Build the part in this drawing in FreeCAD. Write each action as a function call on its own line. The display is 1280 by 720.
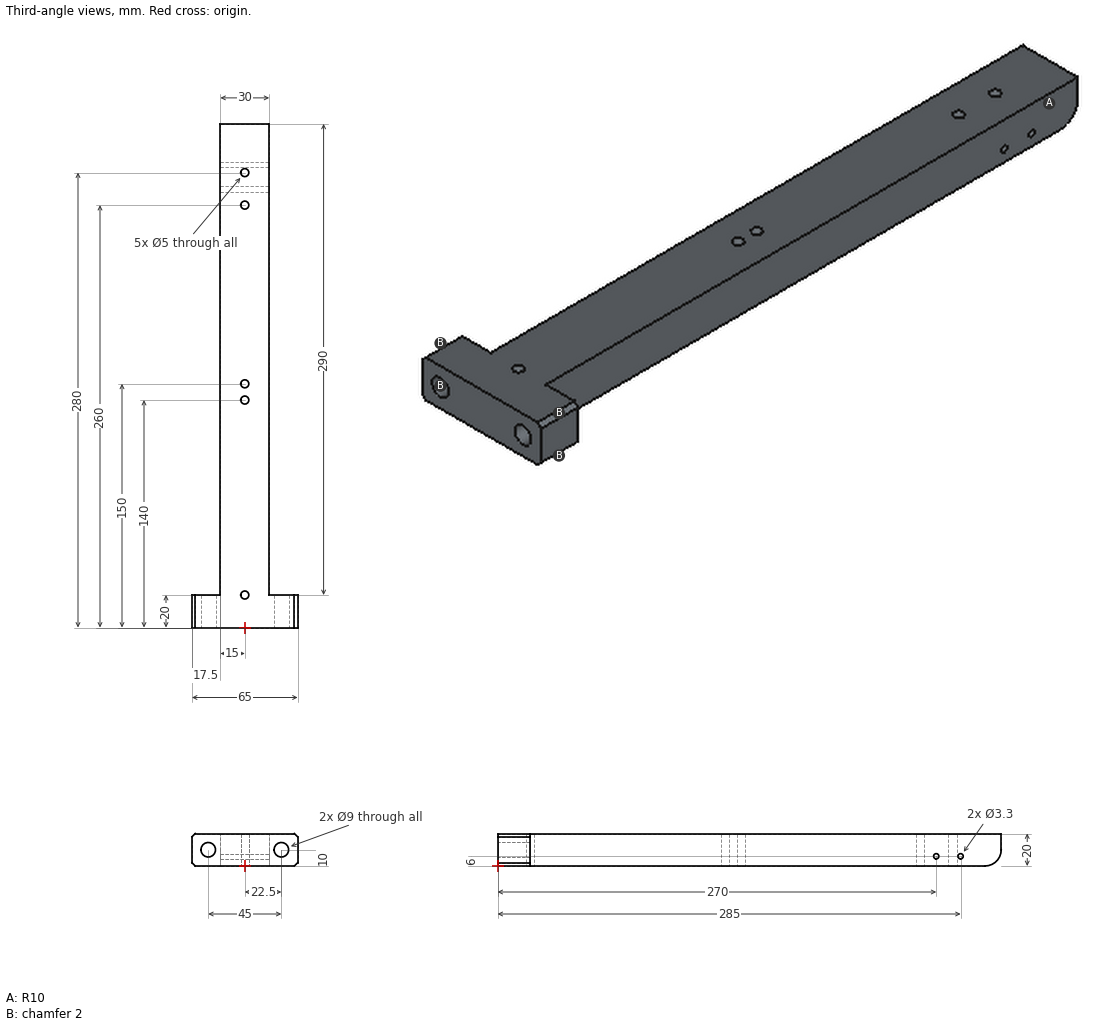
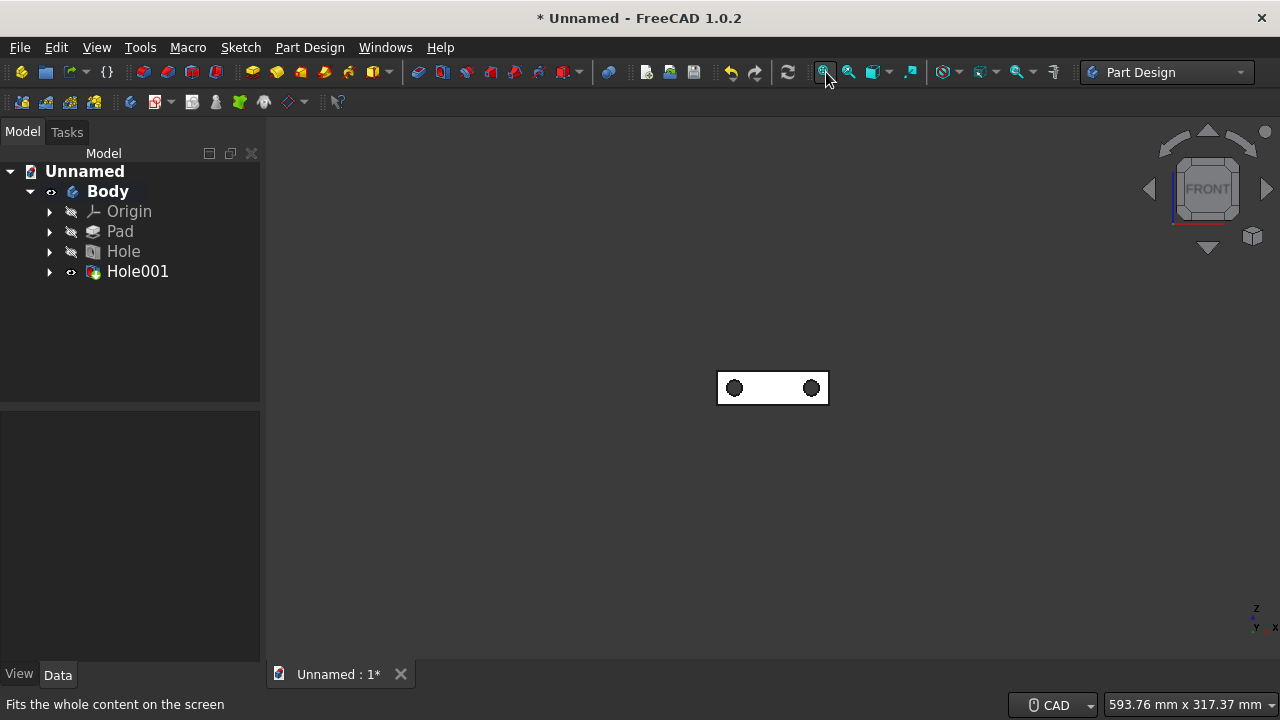
key(3)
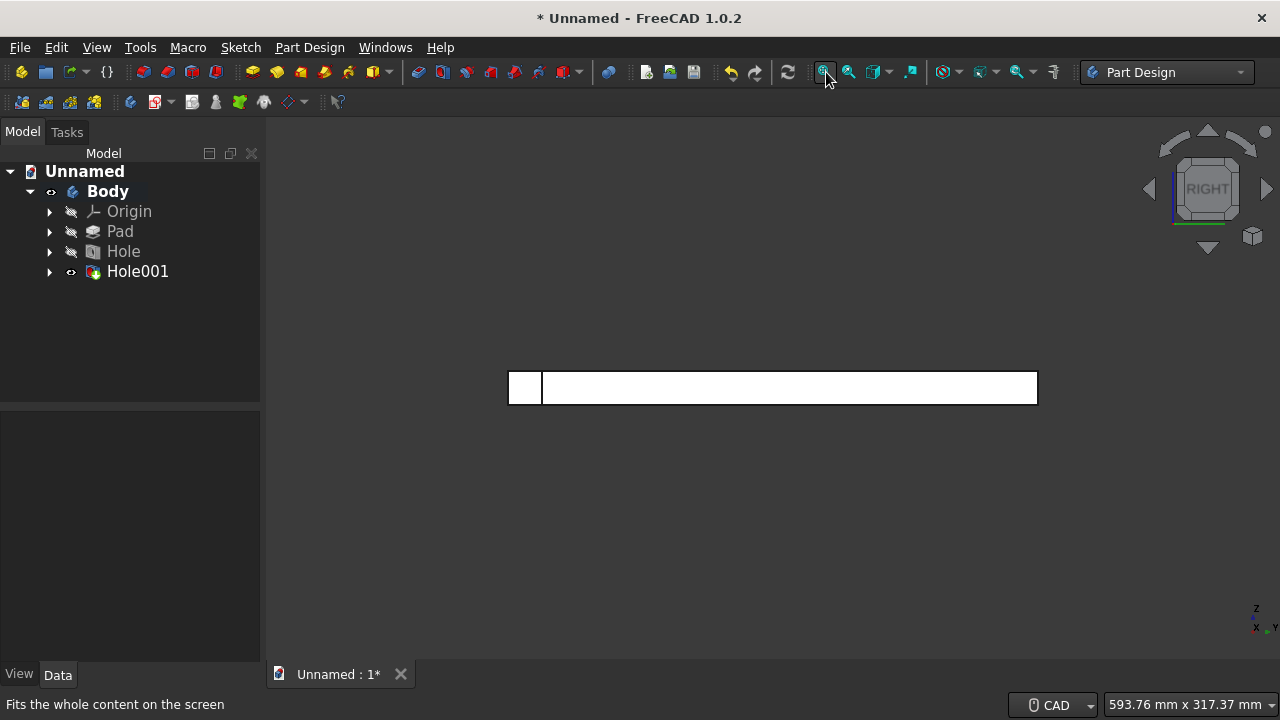
key(5)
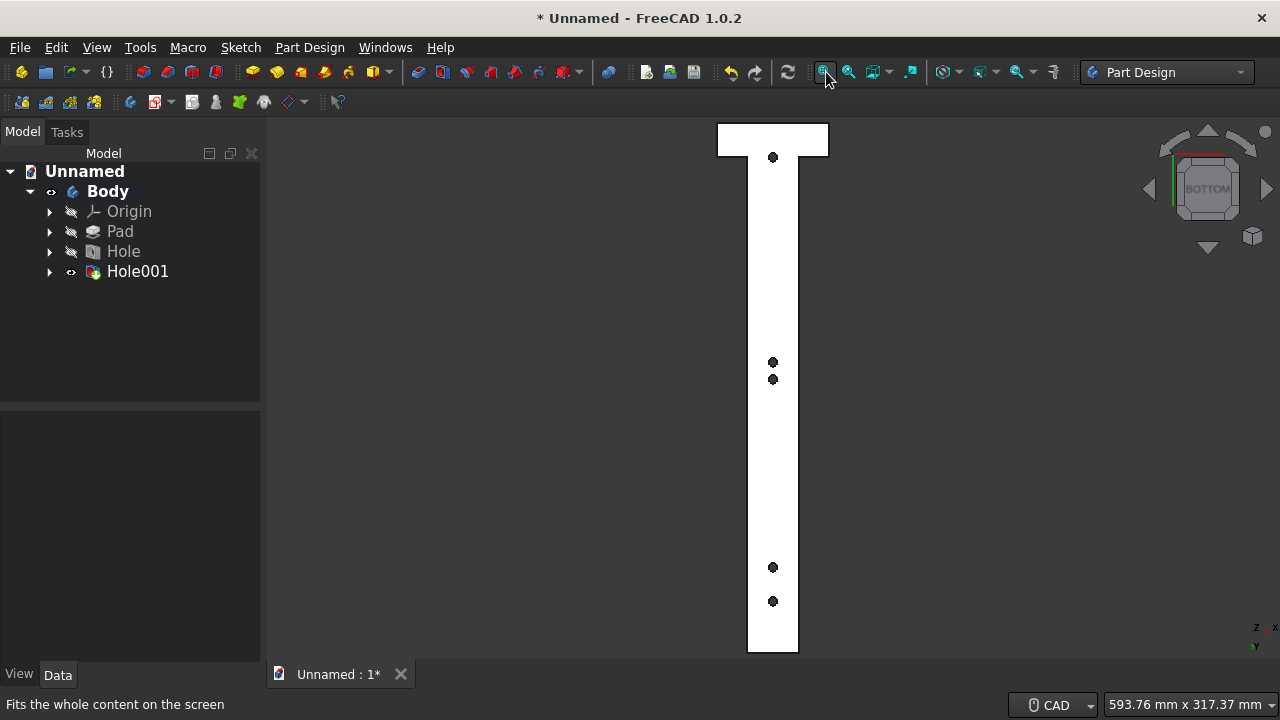
key(4)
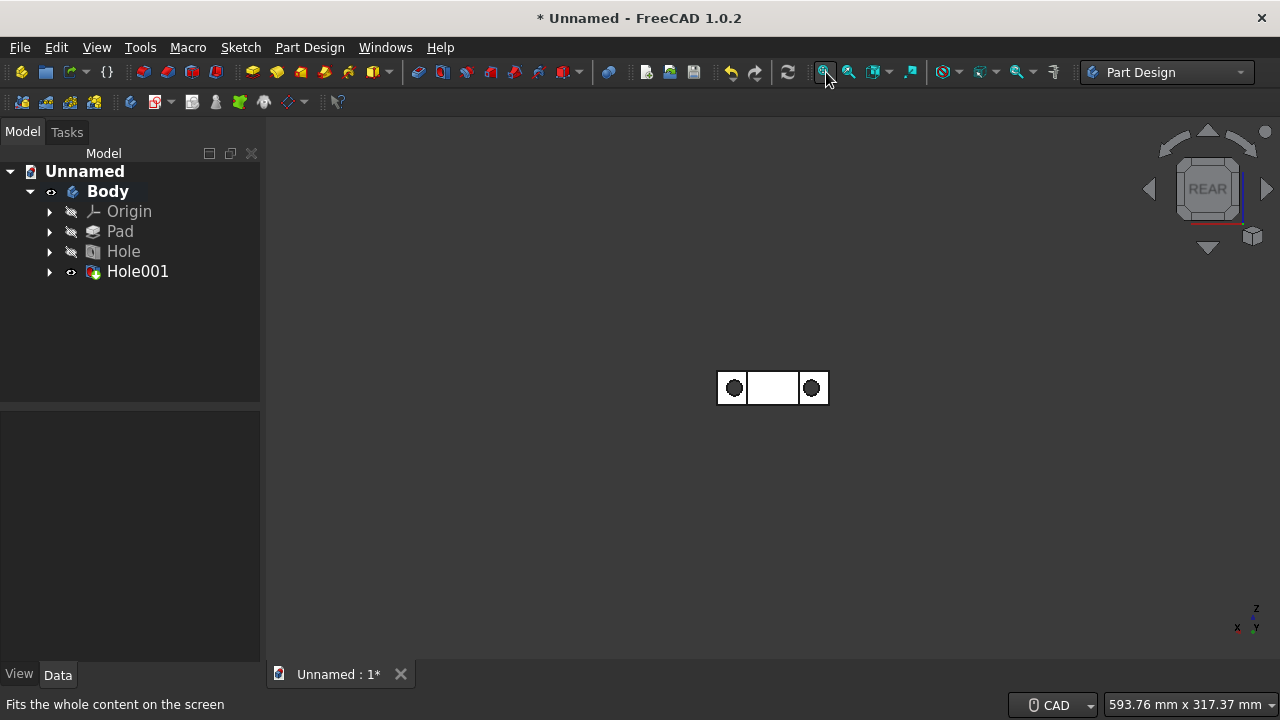
key(v)
key(f)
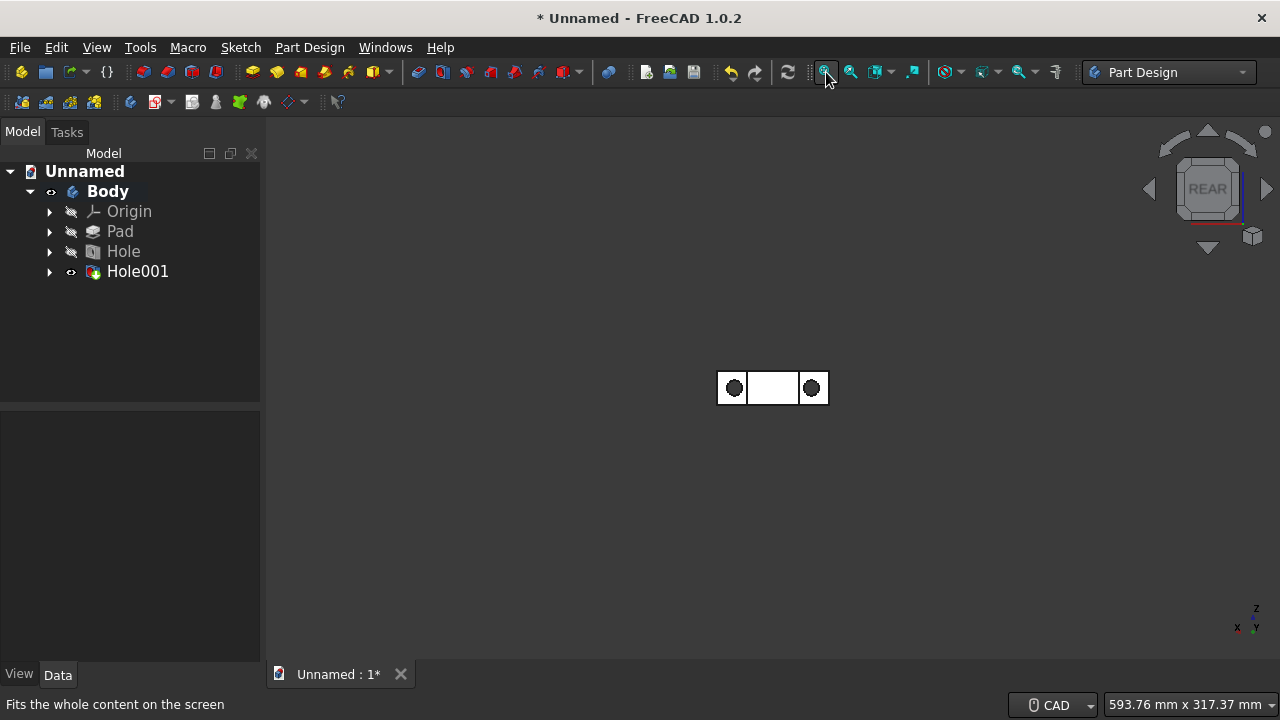
click(773, 404)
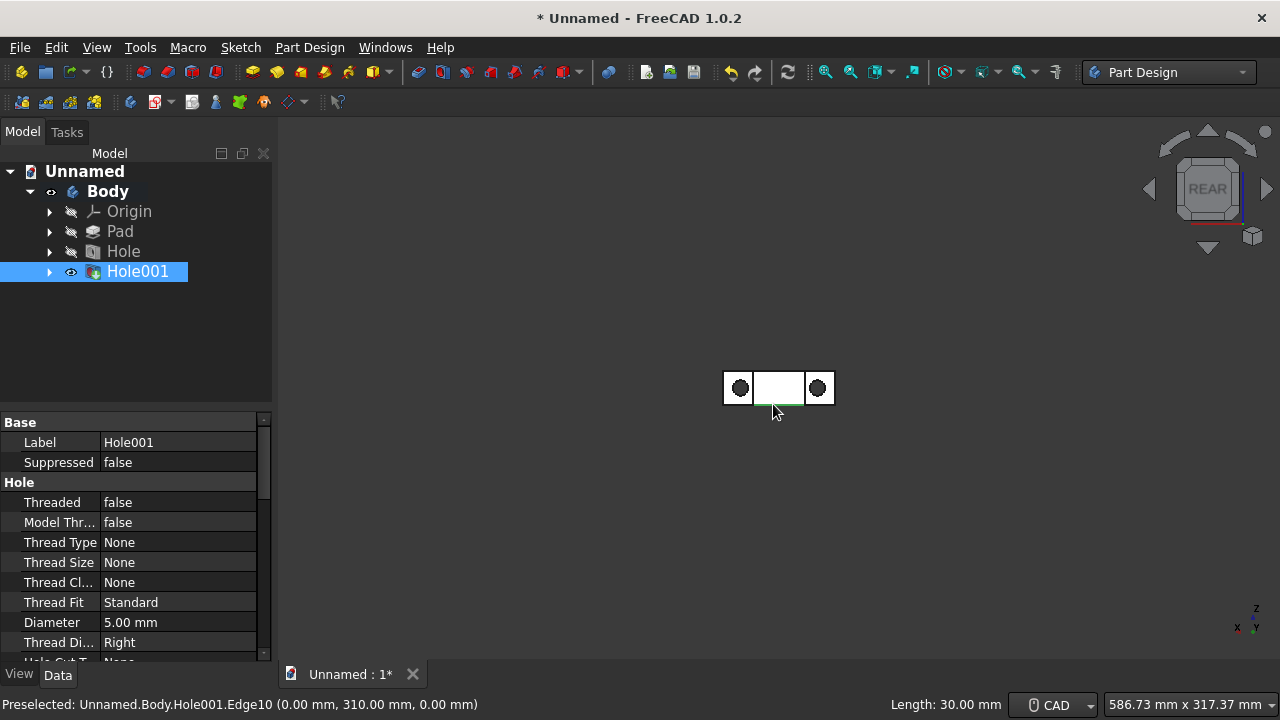
click(144, 72)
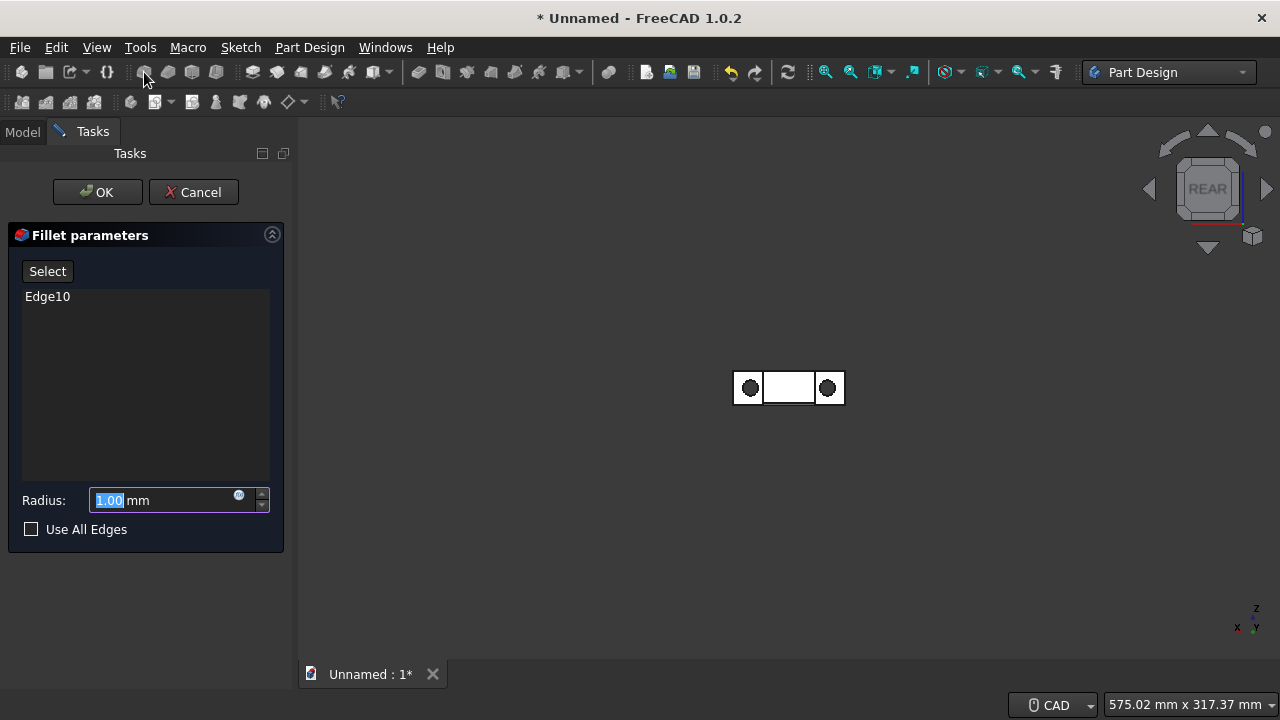
text(10)
key(Tab)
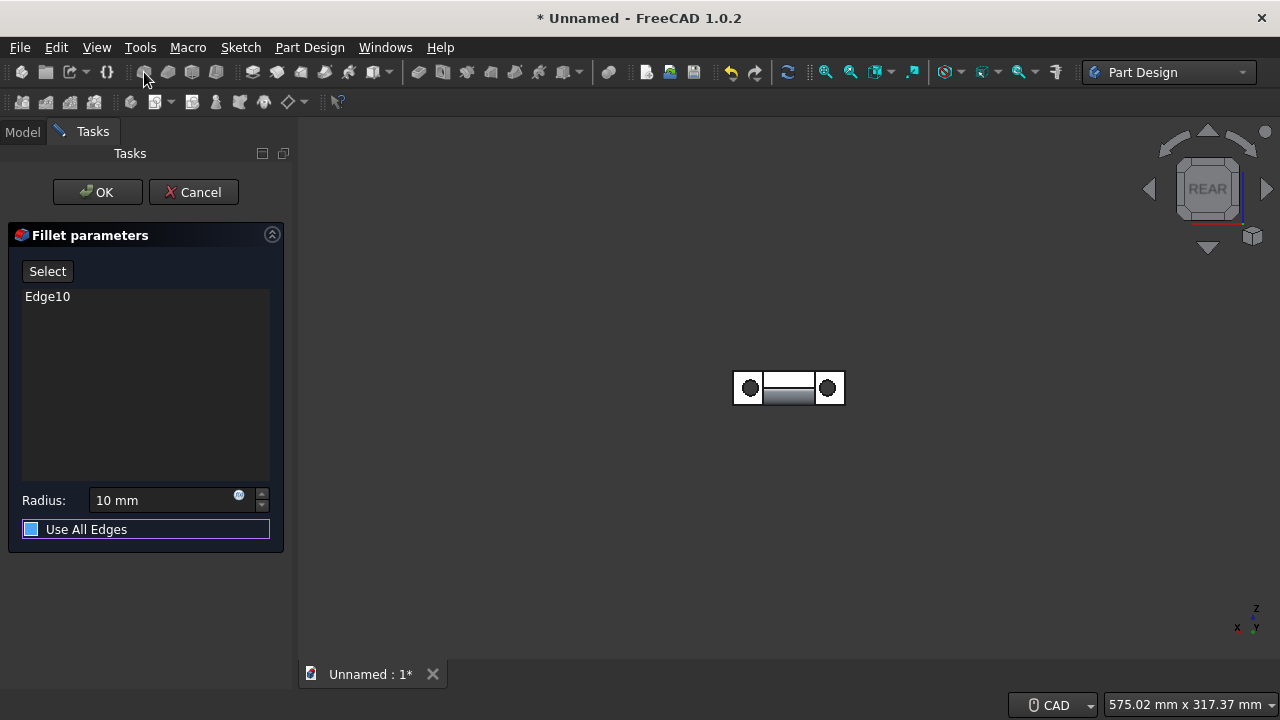
click(98, 192)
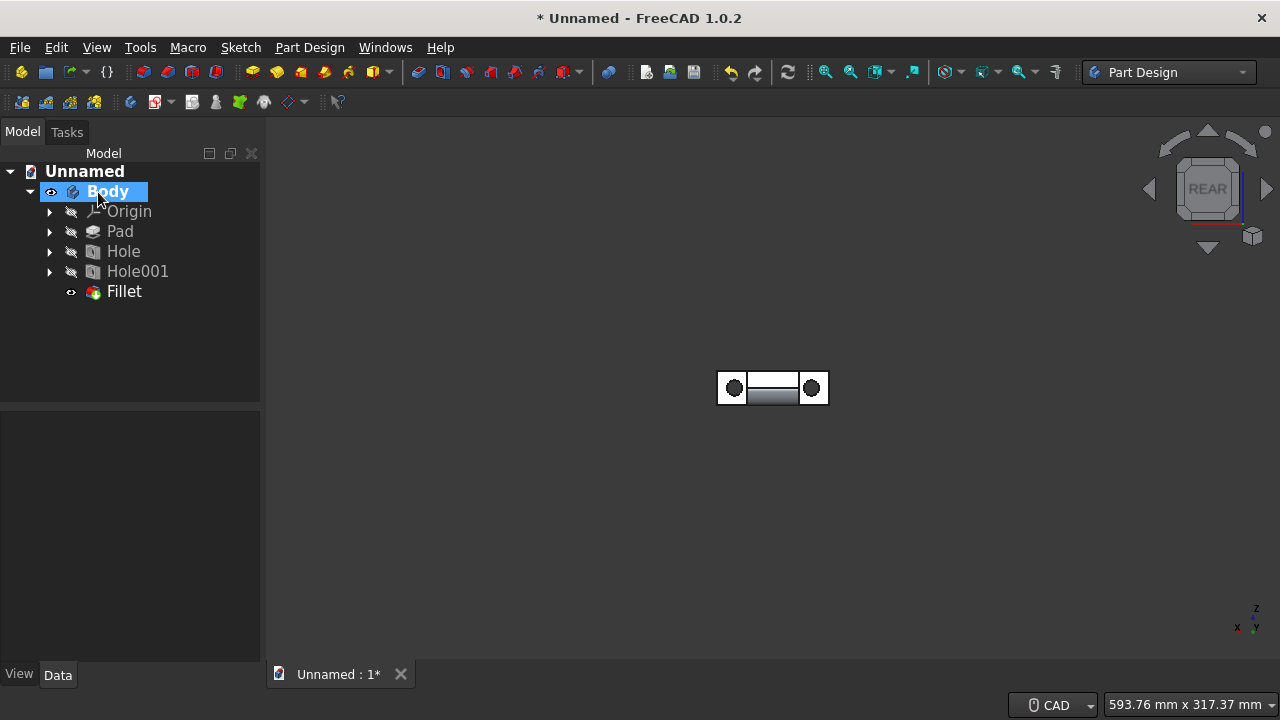
key(v)
key(f)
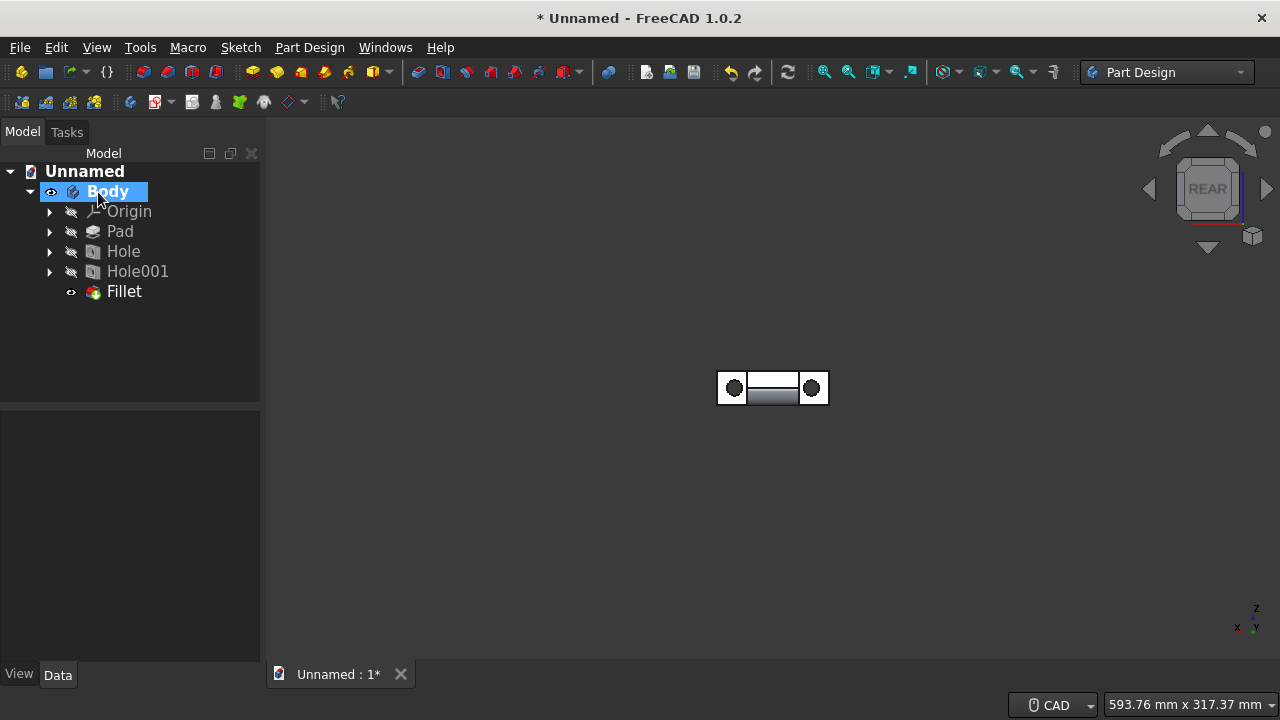
key(0)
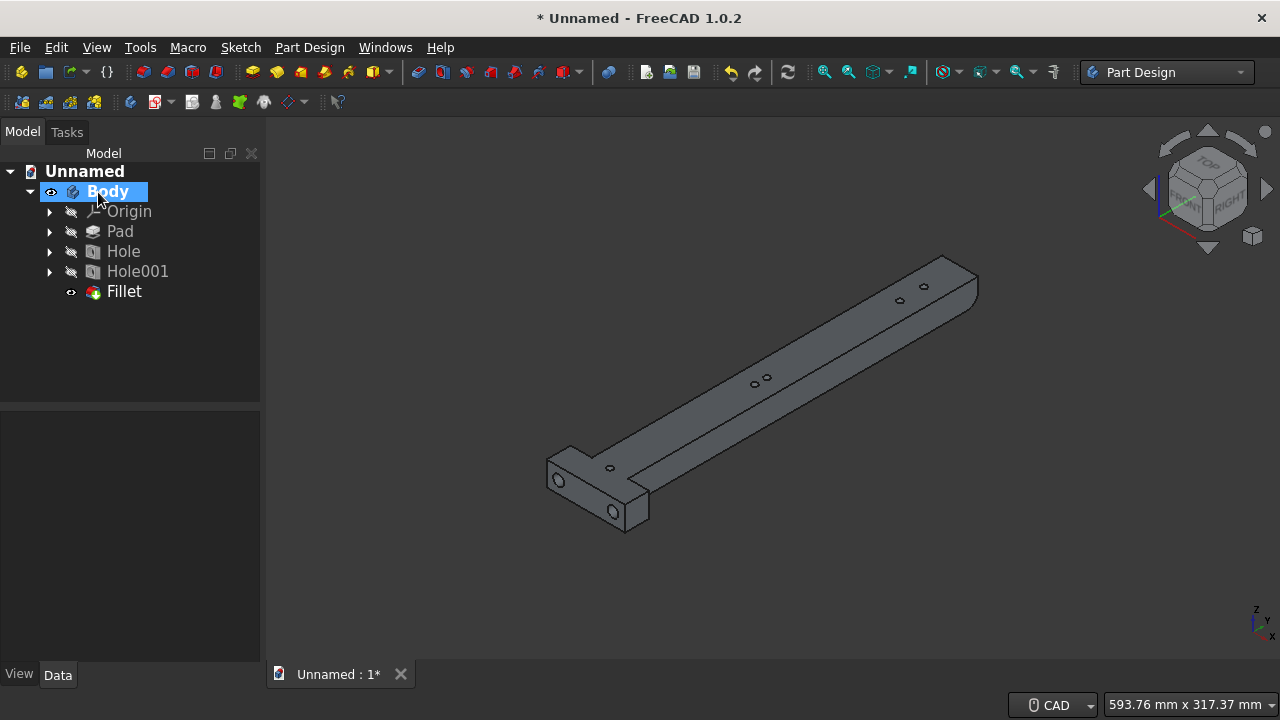
click(637, 497)